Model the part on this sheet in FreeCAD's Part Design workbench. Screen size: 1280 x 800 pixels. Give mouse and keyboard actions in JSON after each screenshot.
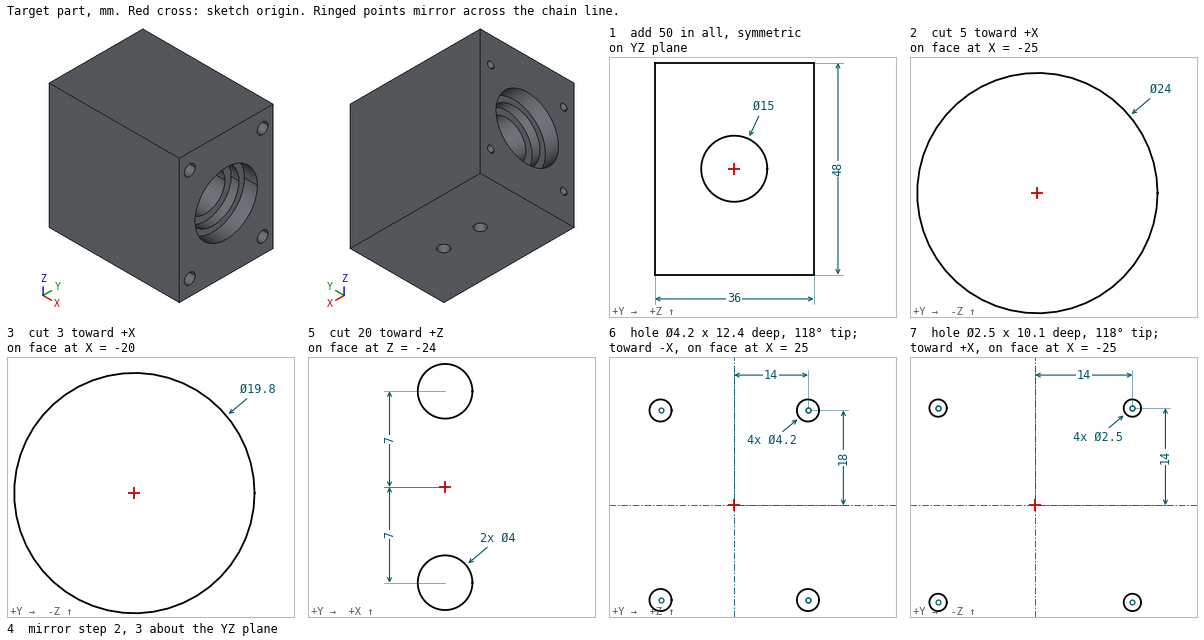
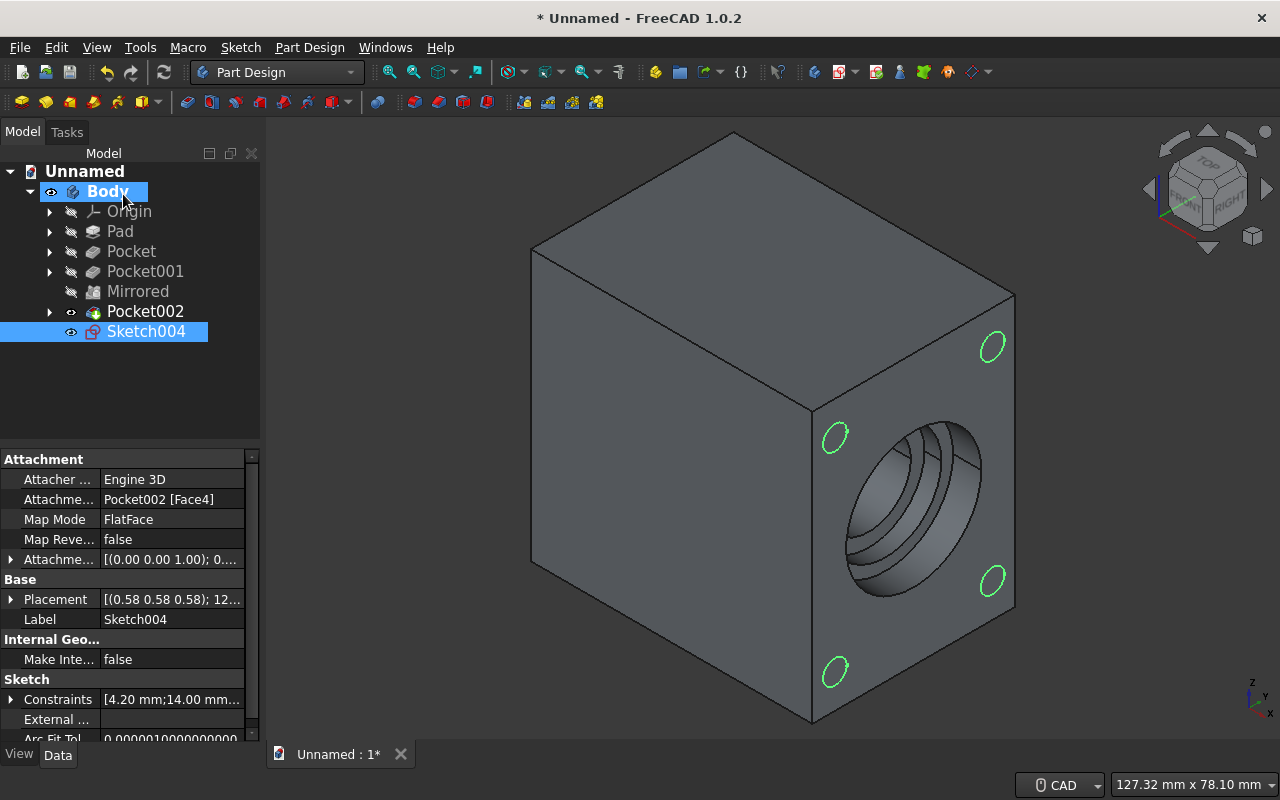
{"action": "left_click", "coordinate": [212, 102]}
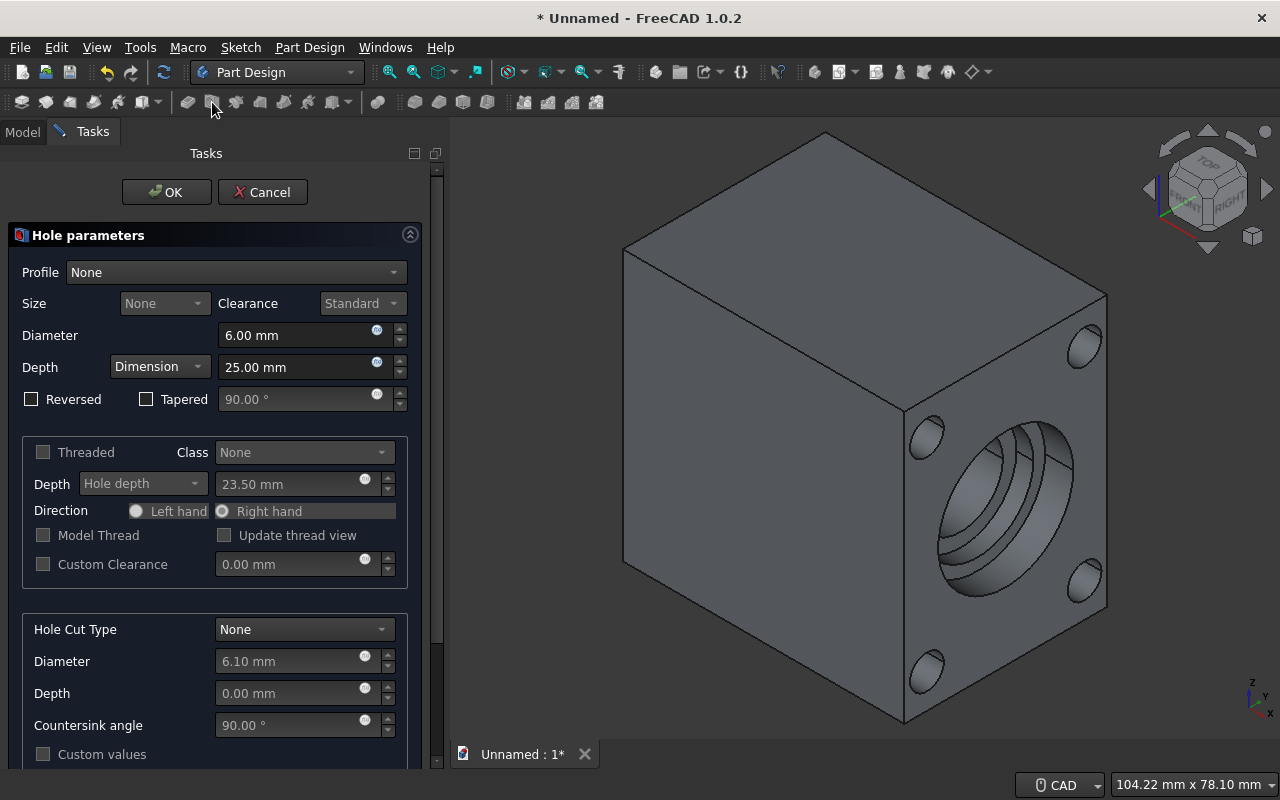
{"action": "triple_click", "coordinate": [305, 335]}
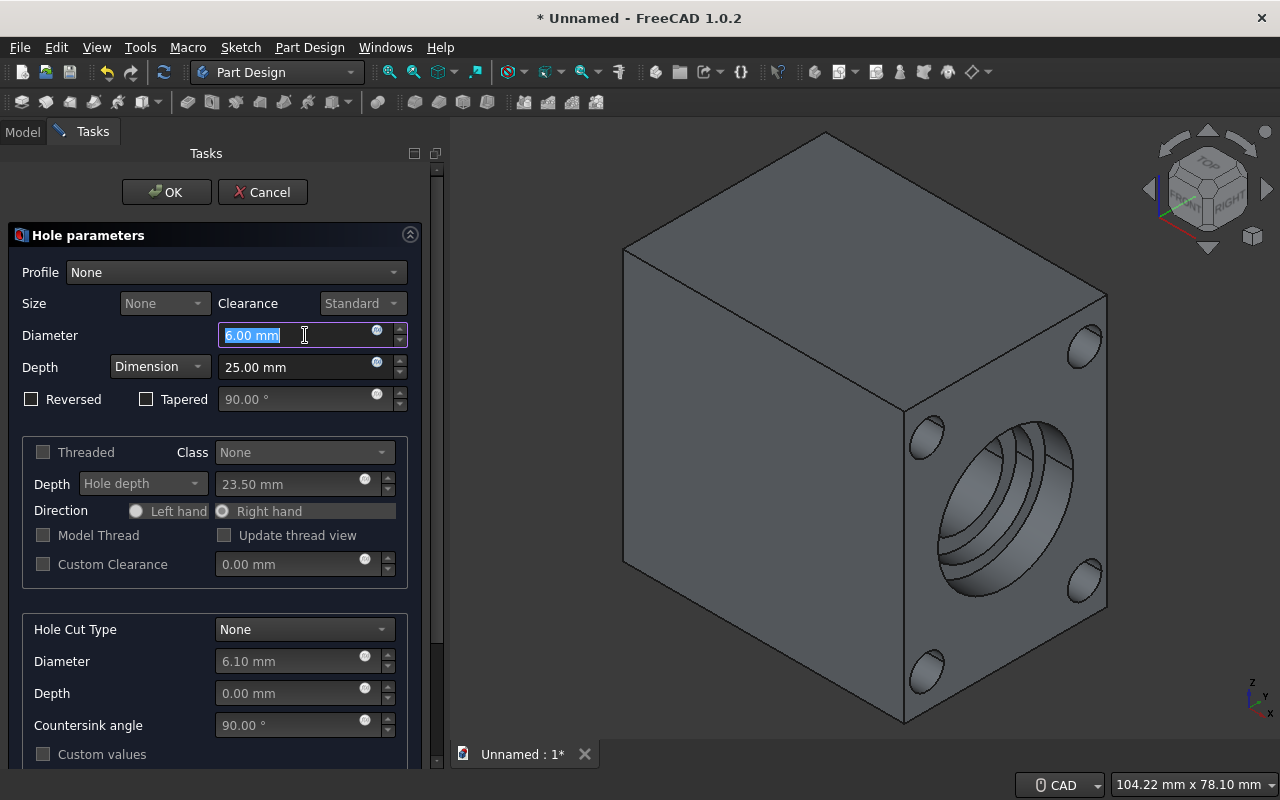
{"action": "type", "text": "4.2"}
{"action": "key", "text": "Tab"}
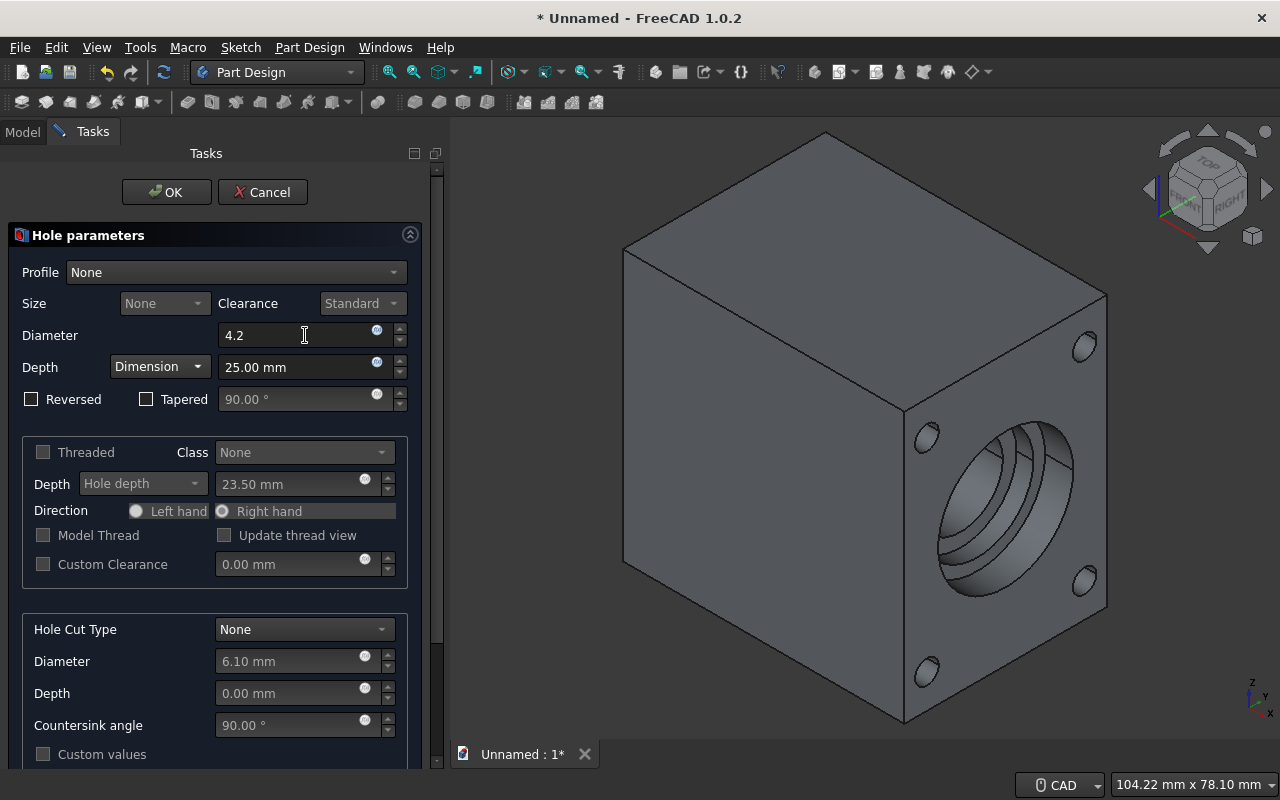
{"action": "triple_click", "coordinate": [305, 367]}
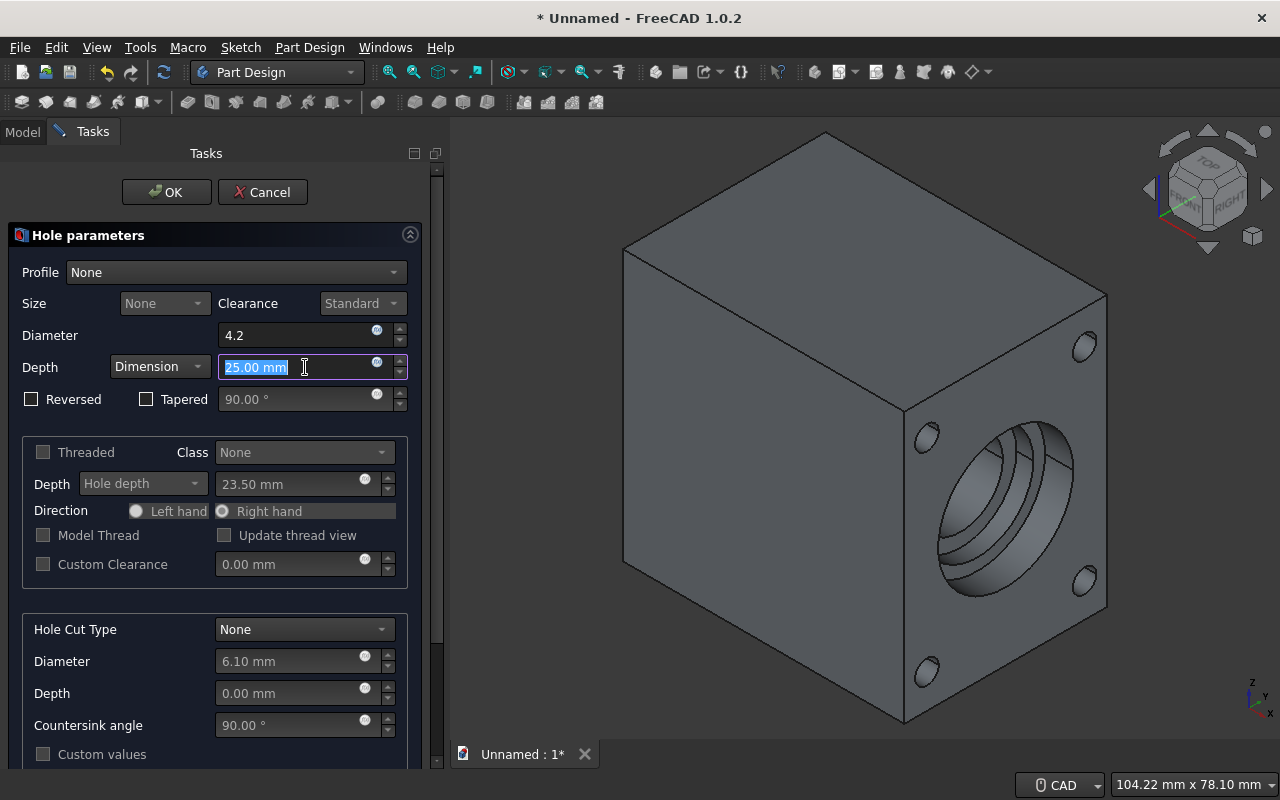
{"action": "type", "text": "12.4"}
{"action": "key", "text": "Tab"}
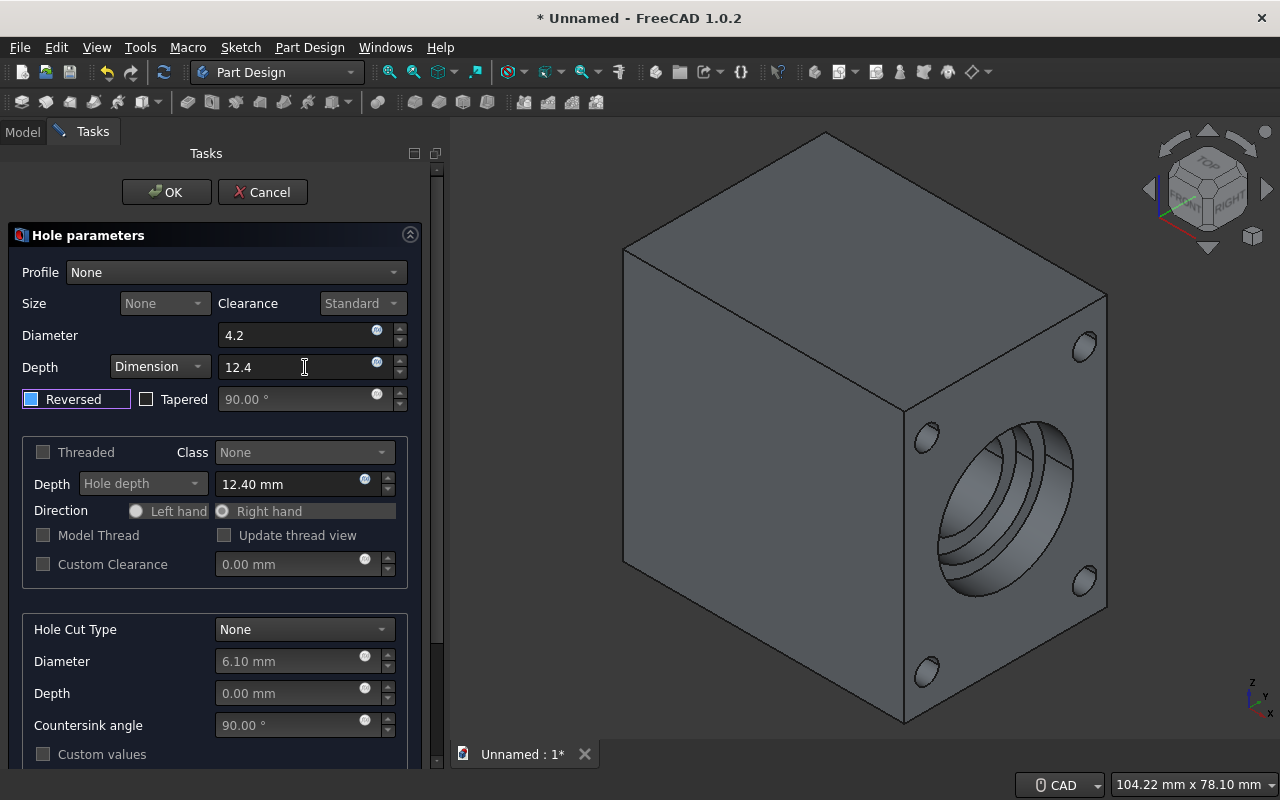
{"action": "left_click", "coordinate": [167, 192]}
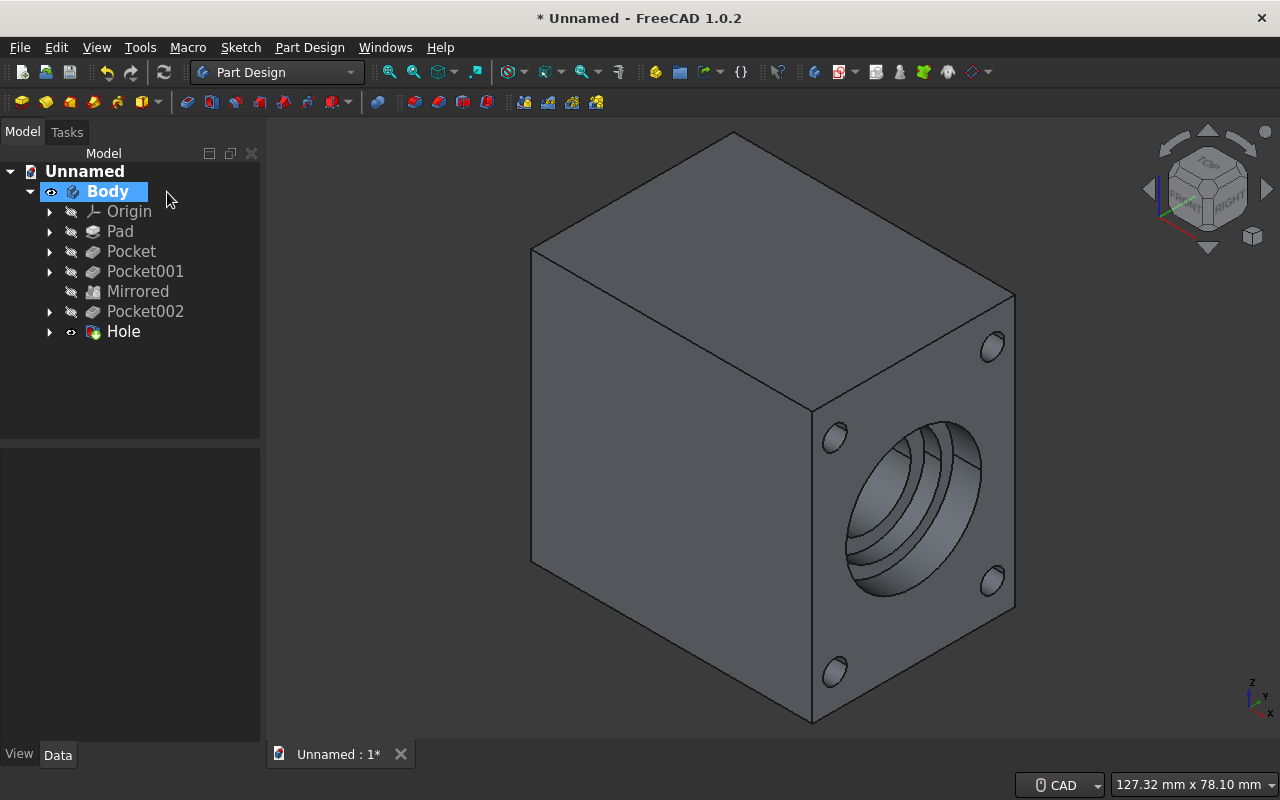
{"action": "key", "text": "6"}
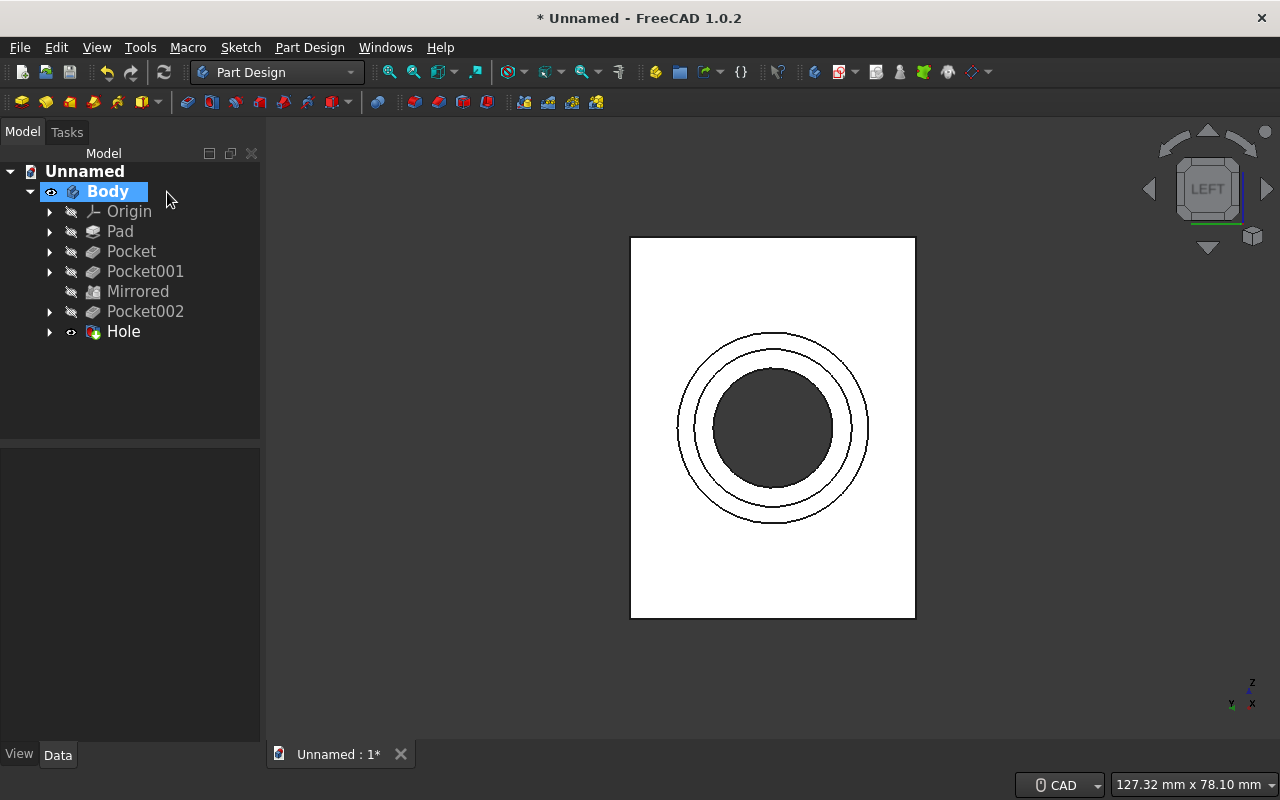
{"action": "left_click", "coordinate": [855, 318]}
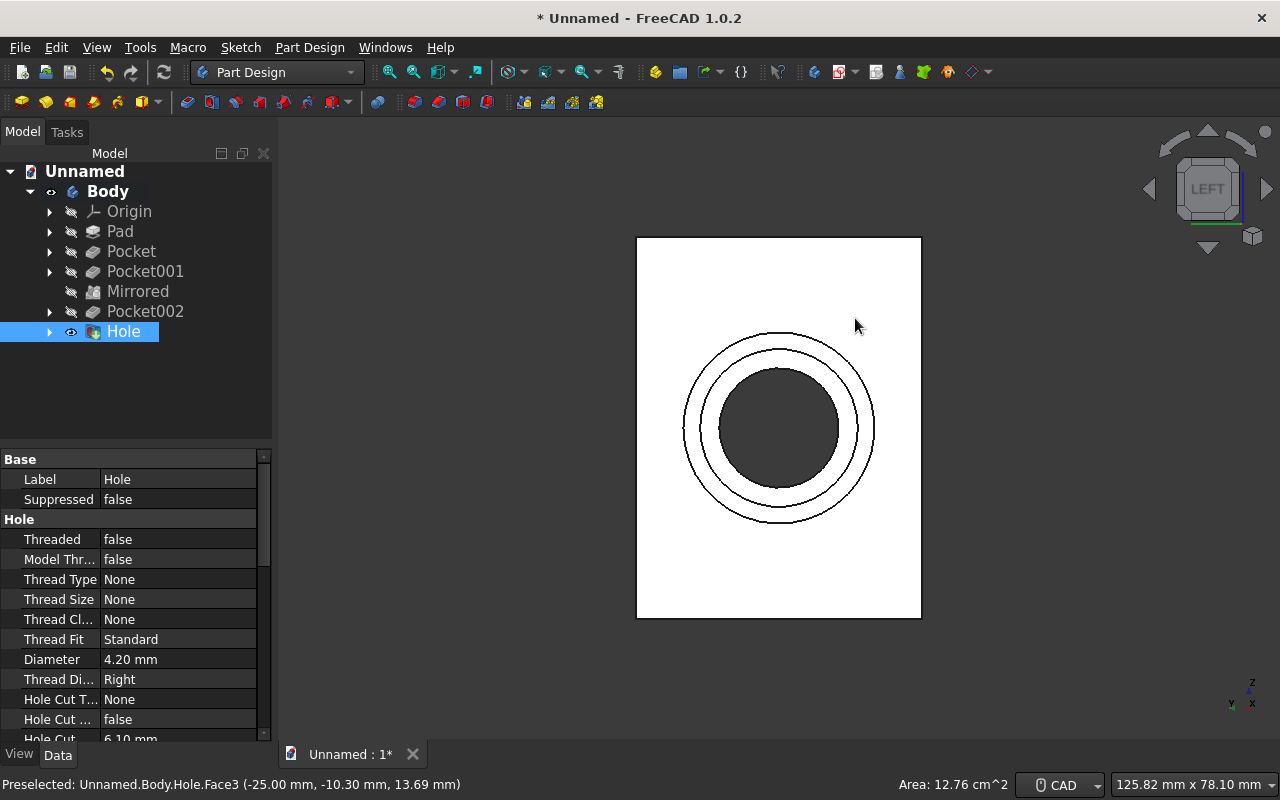
{"action": "left_click", "coordinate": [840, 72]}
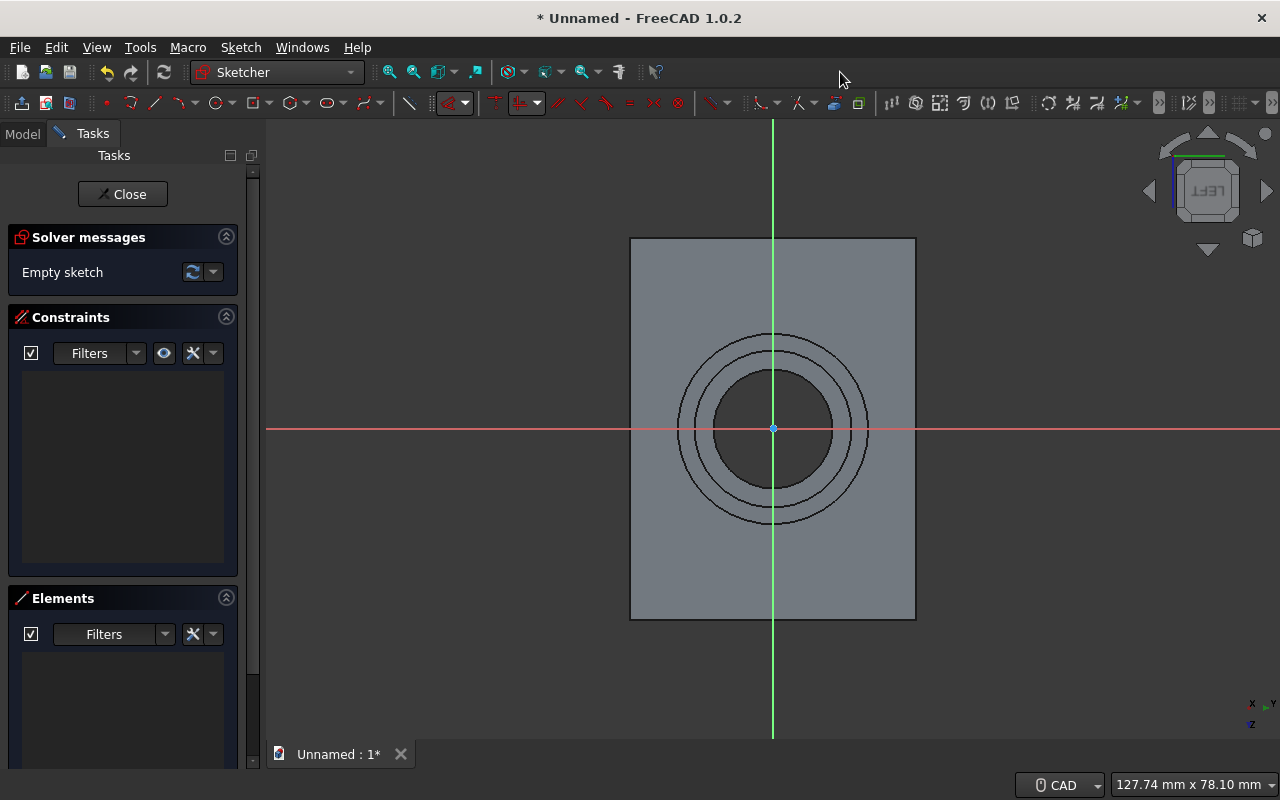
{"action": "scroll", "coordinate": [912, 429], "scroll_direction": "up", "scroll_amount": 2}